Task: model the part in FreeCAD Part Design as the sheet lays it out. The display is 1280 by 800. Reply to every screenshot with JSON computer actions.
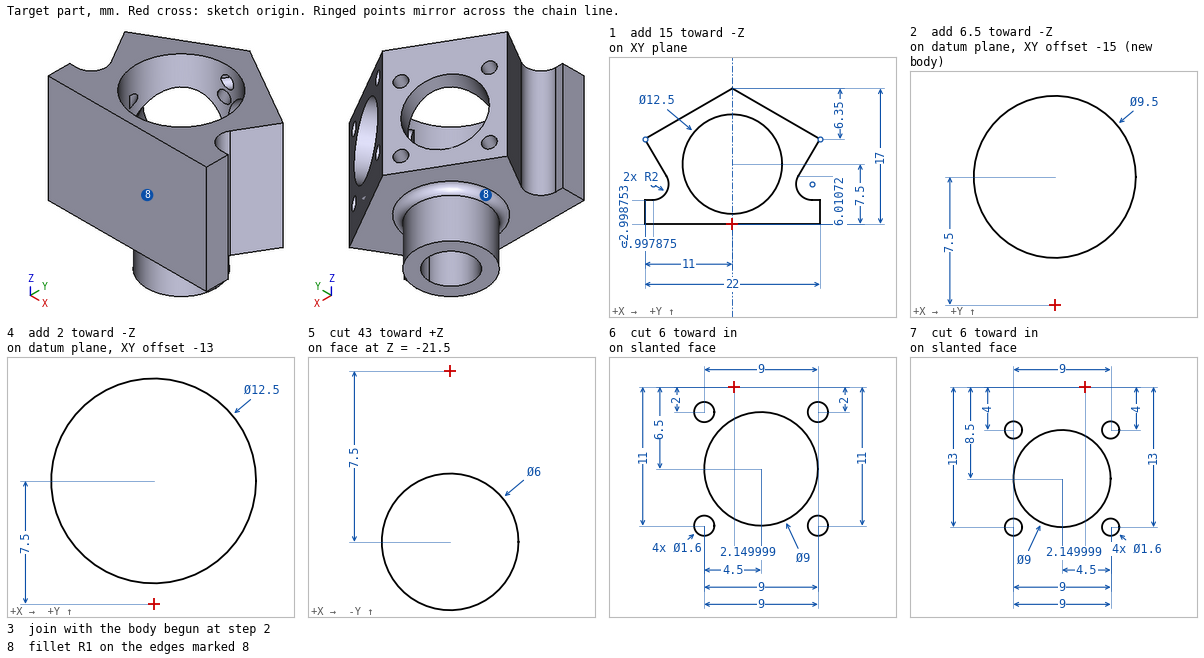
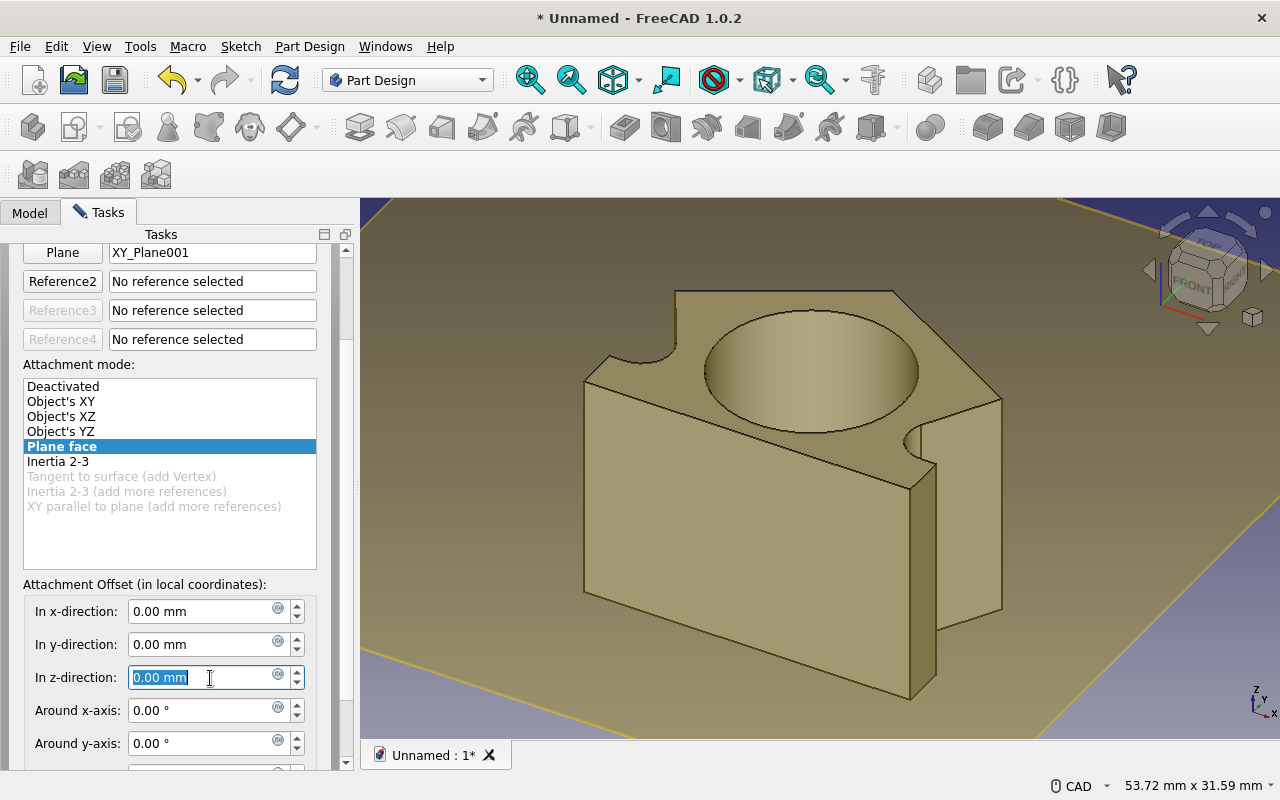
{"action": "type", "text": "-15"}
{"action": "key", "text": "Tab"}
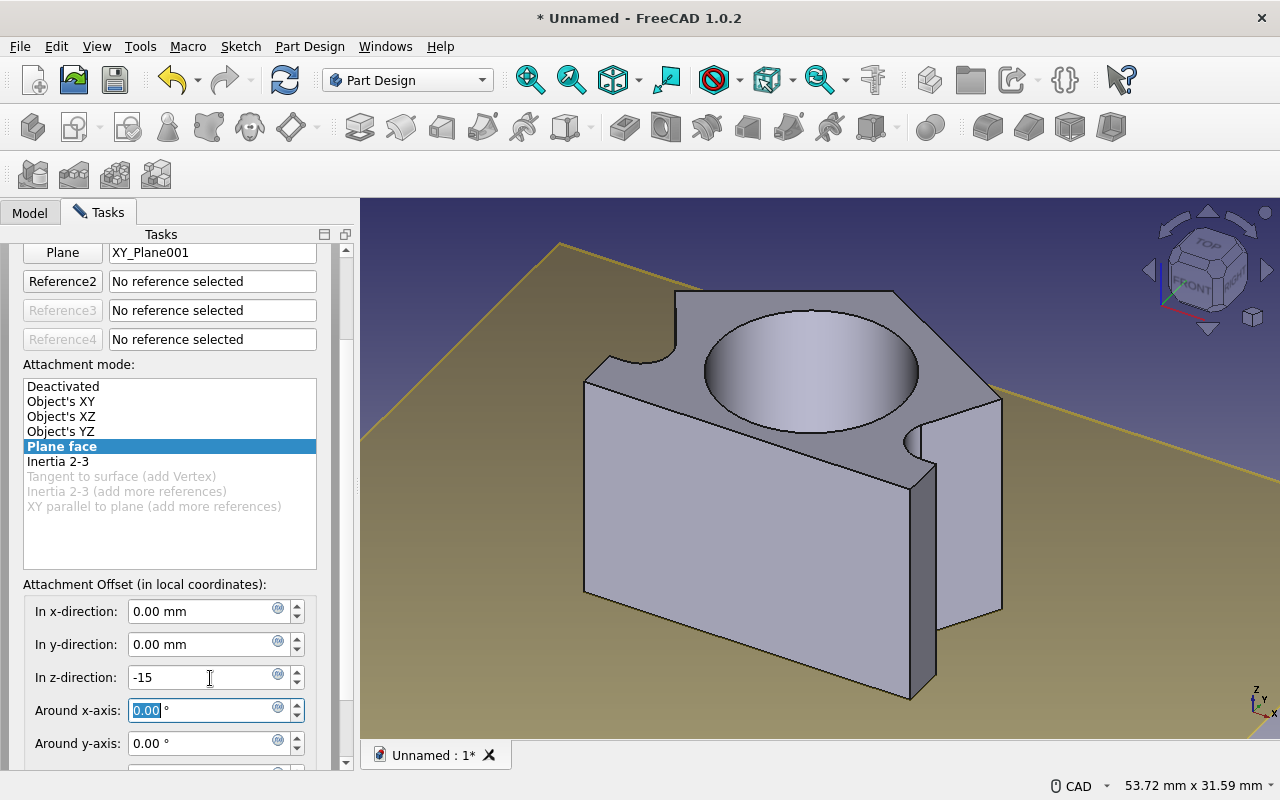
{"action": "scroll", "coordinate": [346, 507], "scroll_direction": "up", "scroll_amount": 3}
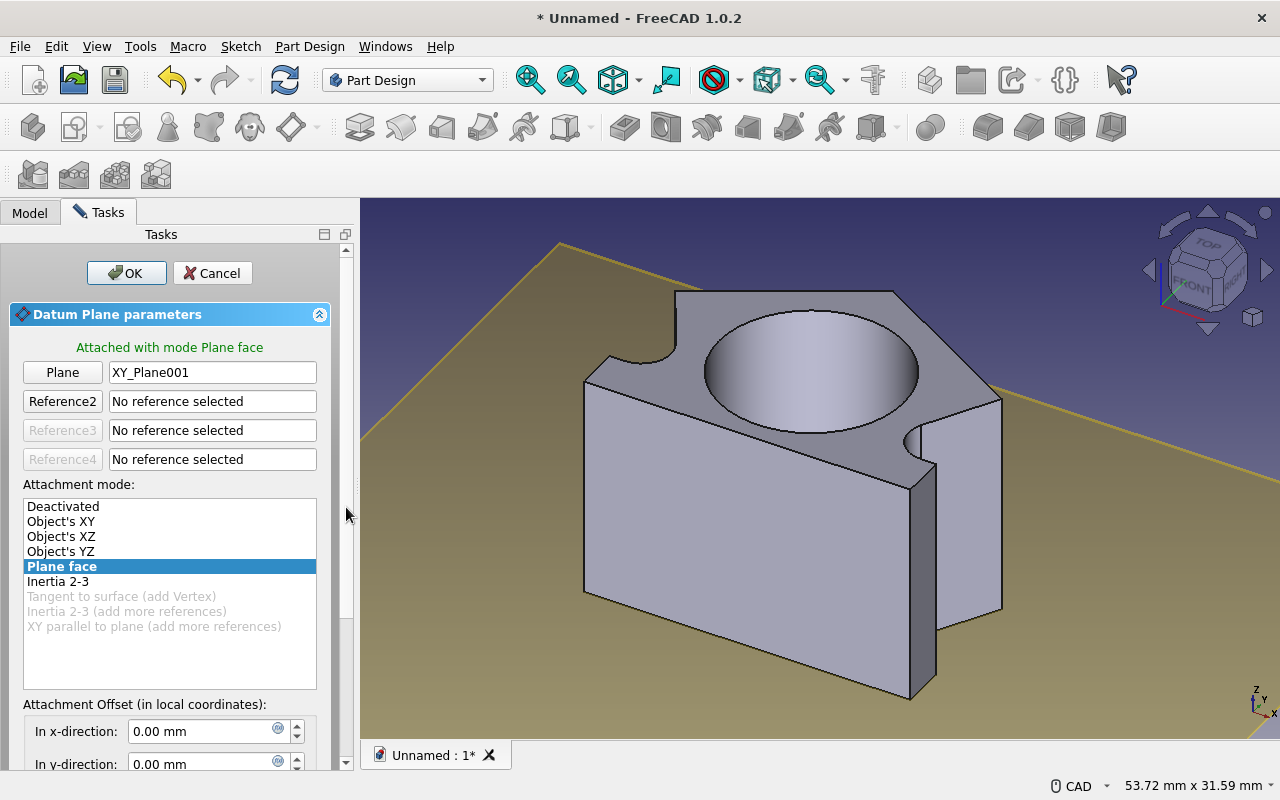
{"action": "left_click", "coordinate": [127, 273]}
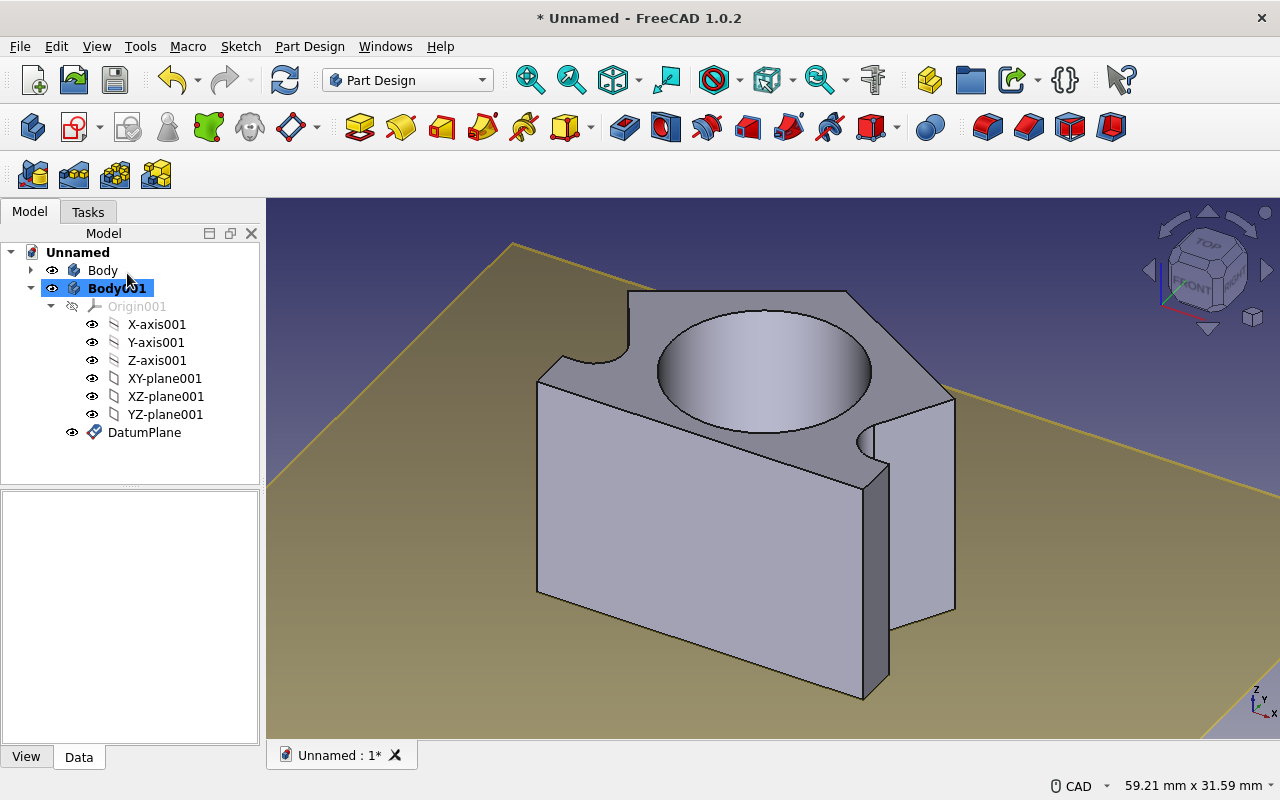
{"action": "left_click", "coordinate": [117, 432]}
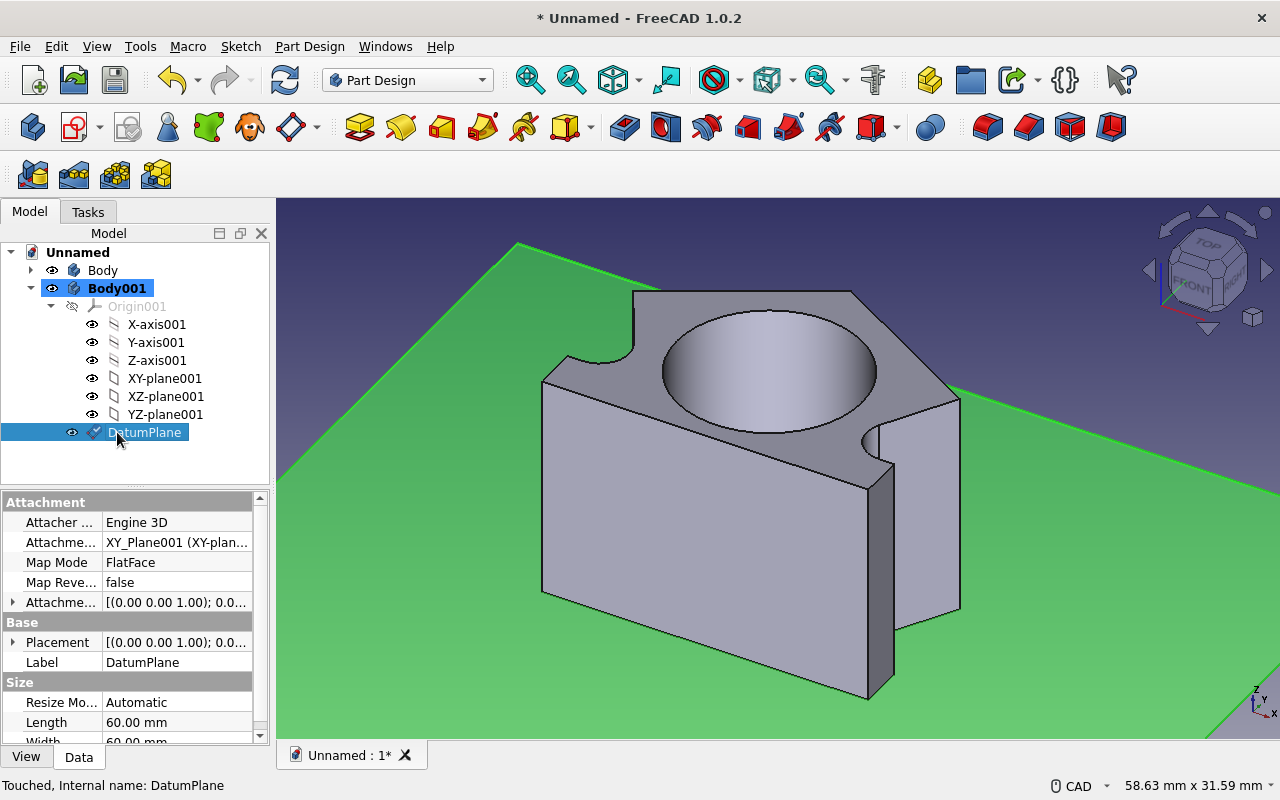
{"action": "left_click", "coordinate": [74, 128]}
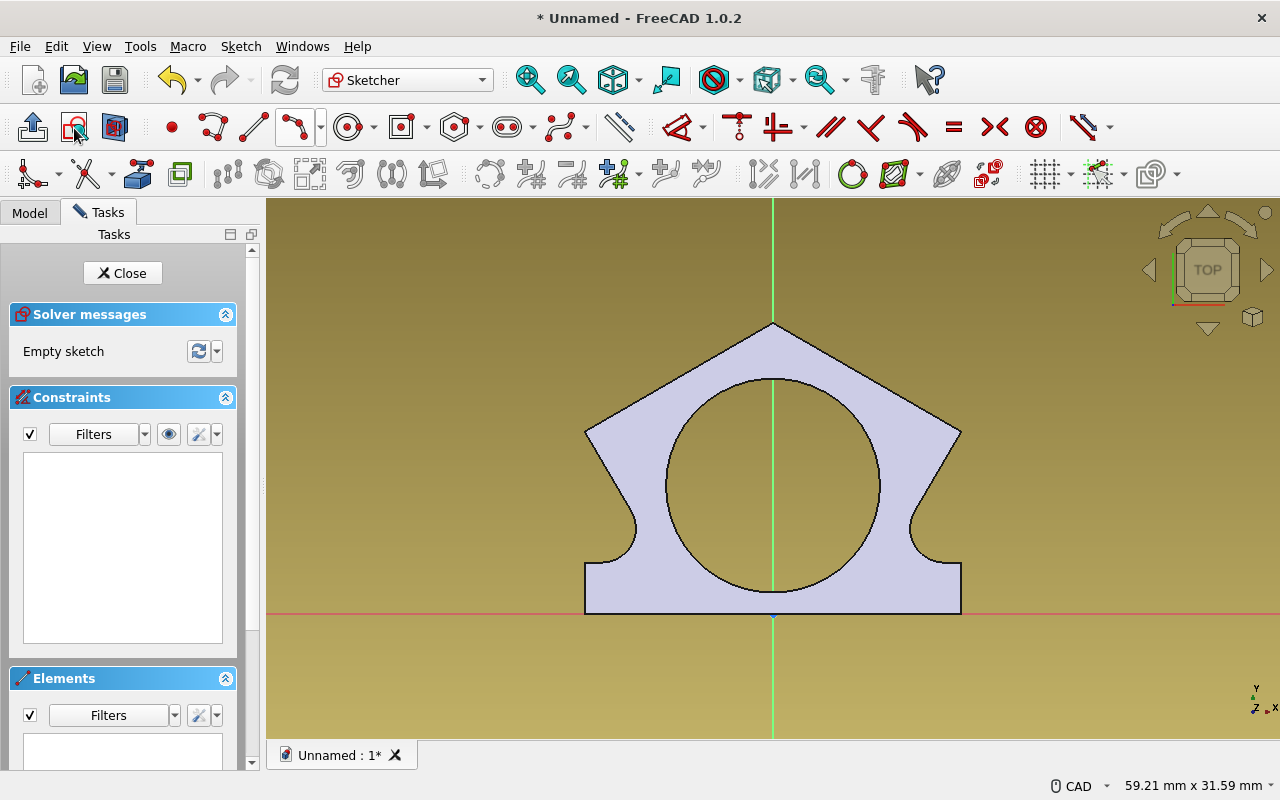
{"action": "scroll", "coordinate": [912, 592], "scroll_direction": "up", "scroll_amount": 2}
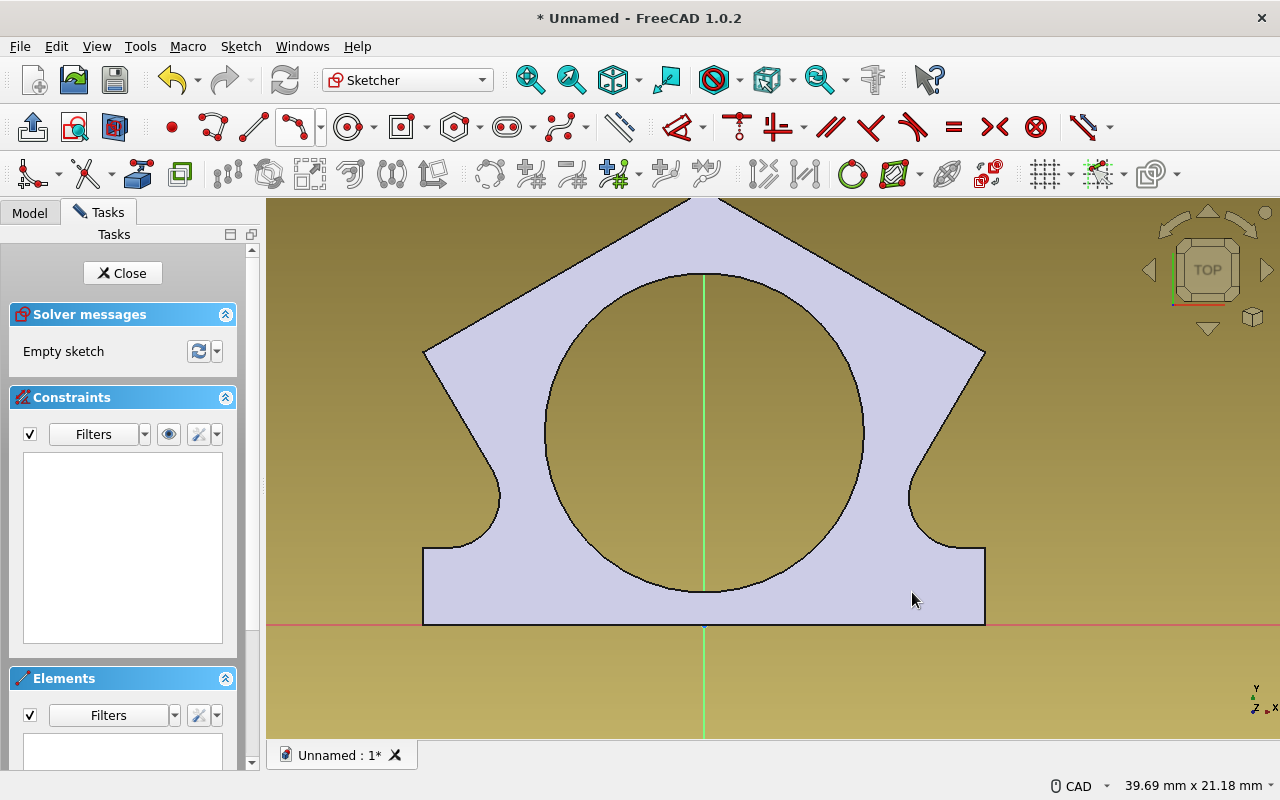
{"action": "left_click", "coordinate": [348, 128]}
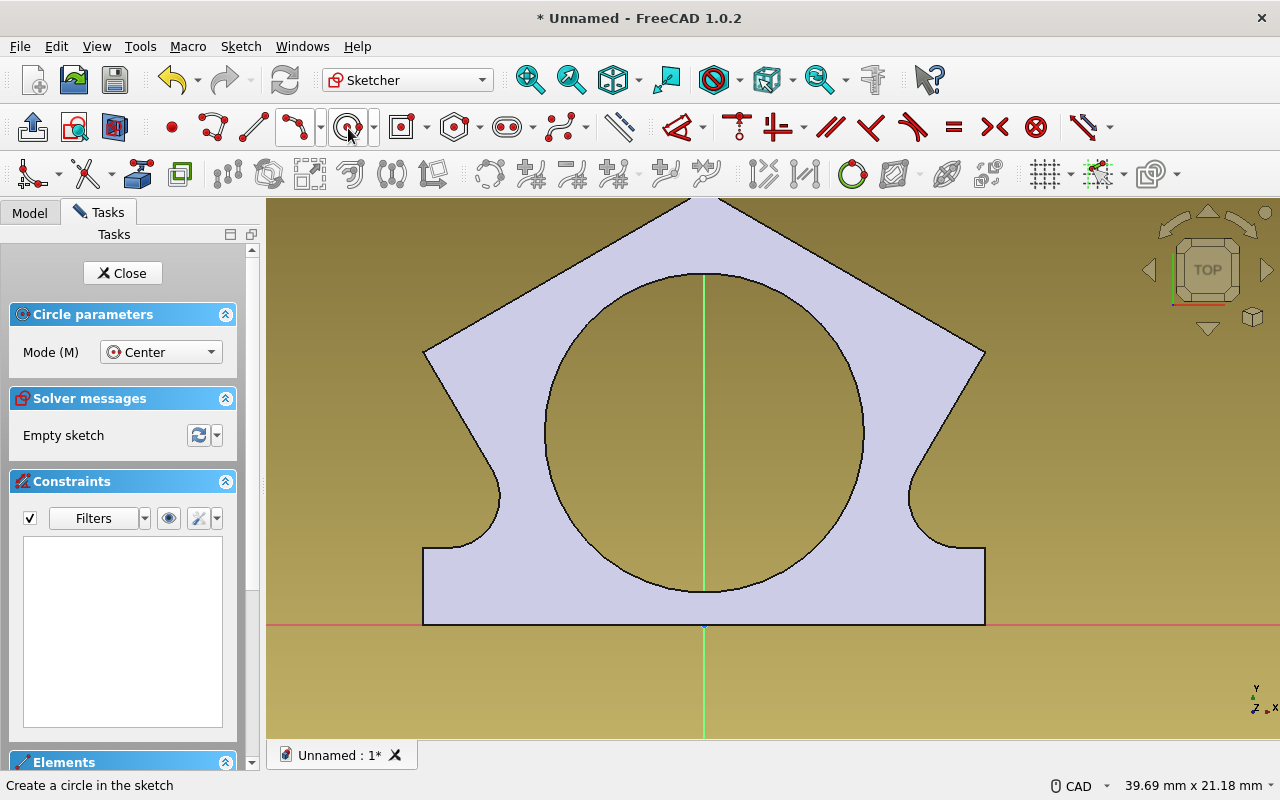
{"action": "left_click", "coordinate": [704, 433]}
{"action": "mouse_move", "coordinate": [790, 347]}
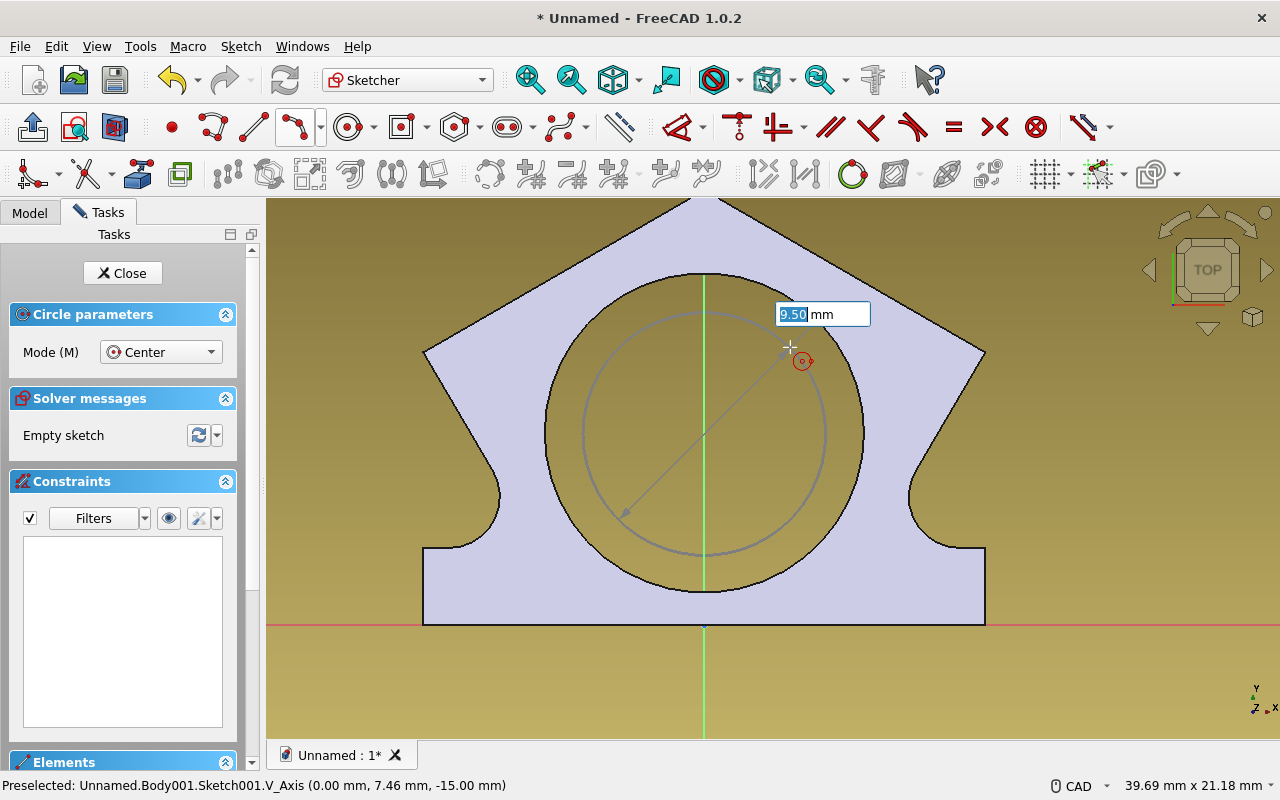
{"action": "type", "text": "9.5"}
{"action": "key", "text": "Return"}
{"action": "key", "text": "Escape"}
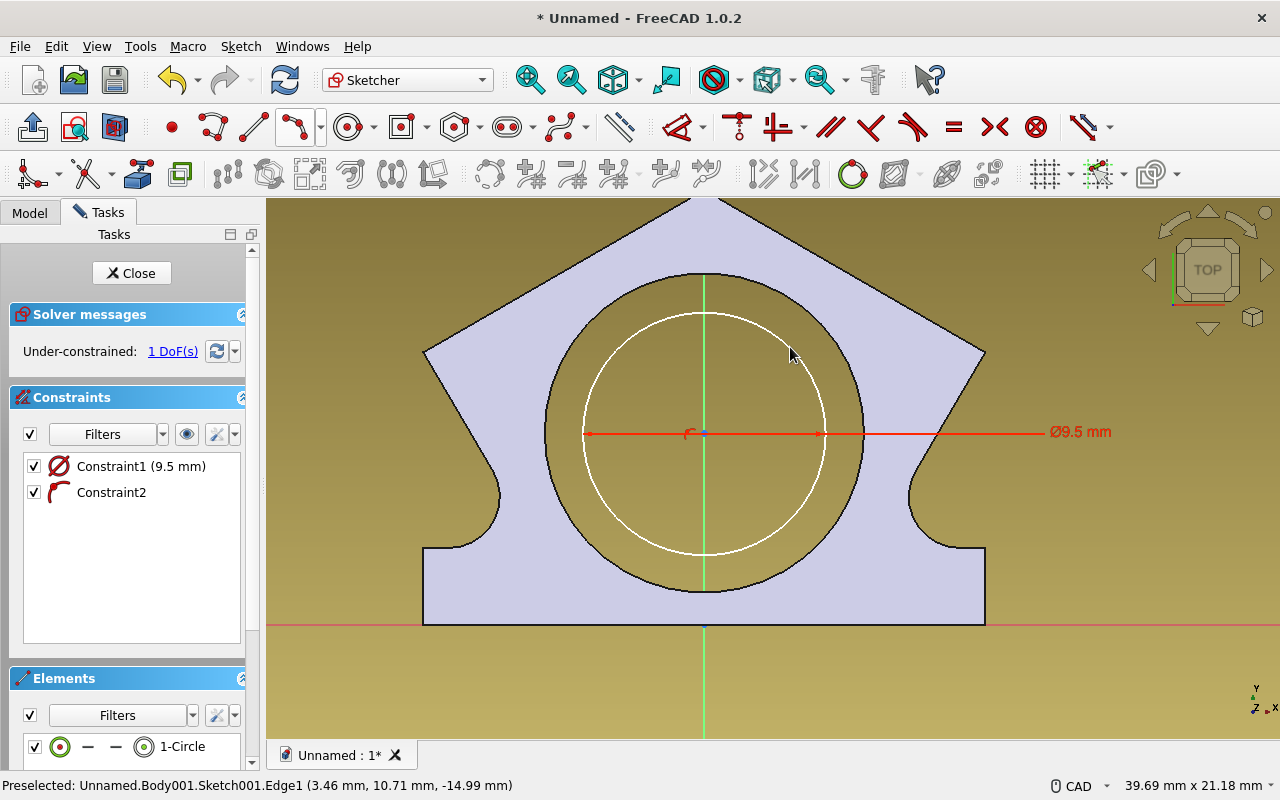
{"action": "left_click", "coordinate": [676, 128]}